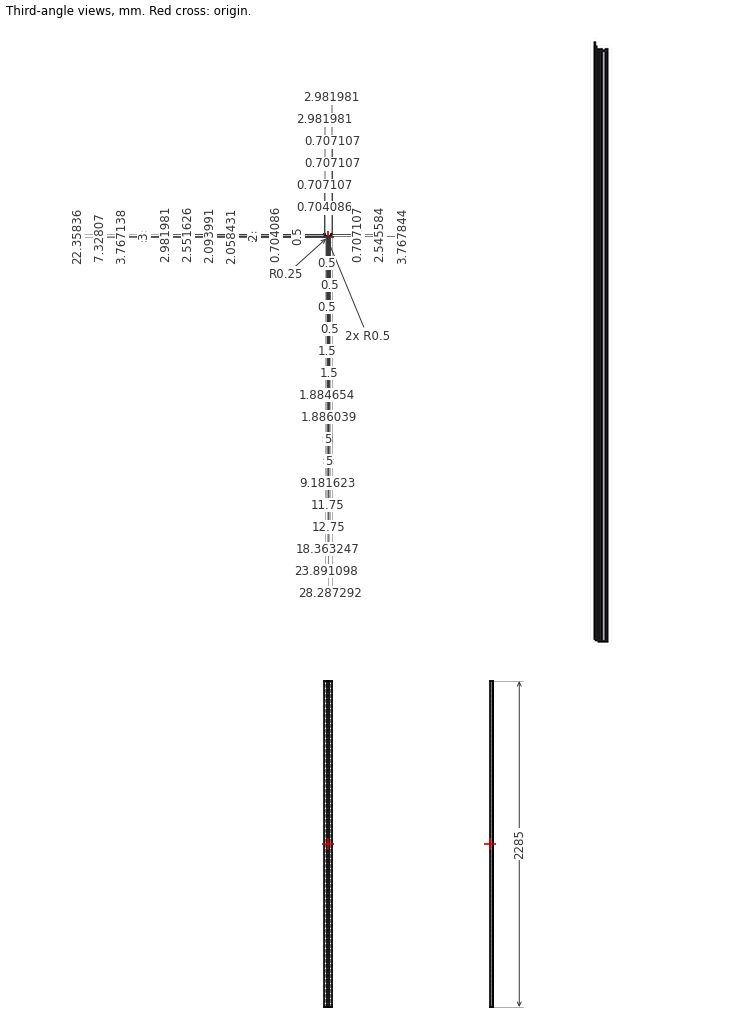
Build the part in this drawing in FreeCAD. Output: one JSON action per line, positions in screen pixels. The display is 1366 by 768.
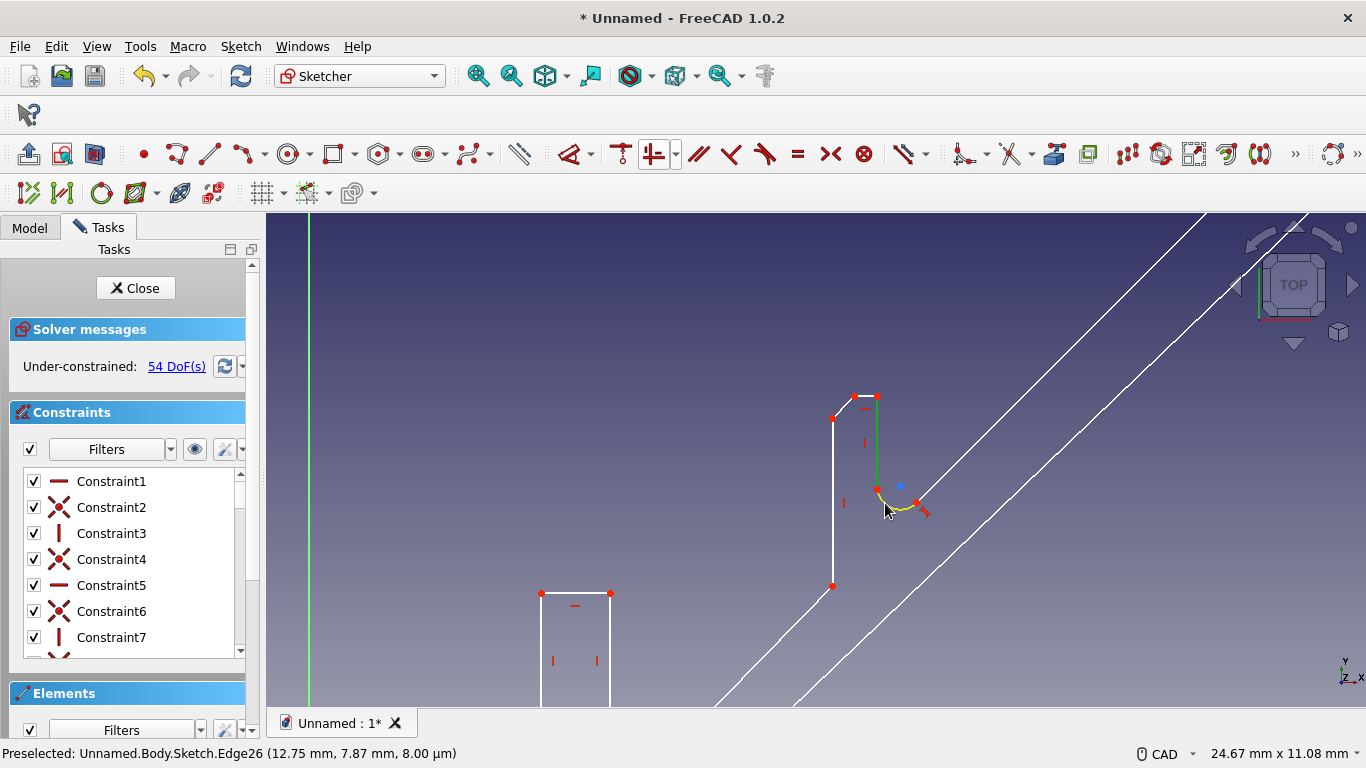
{"action": "left_click", "coordinate": [884, 503]}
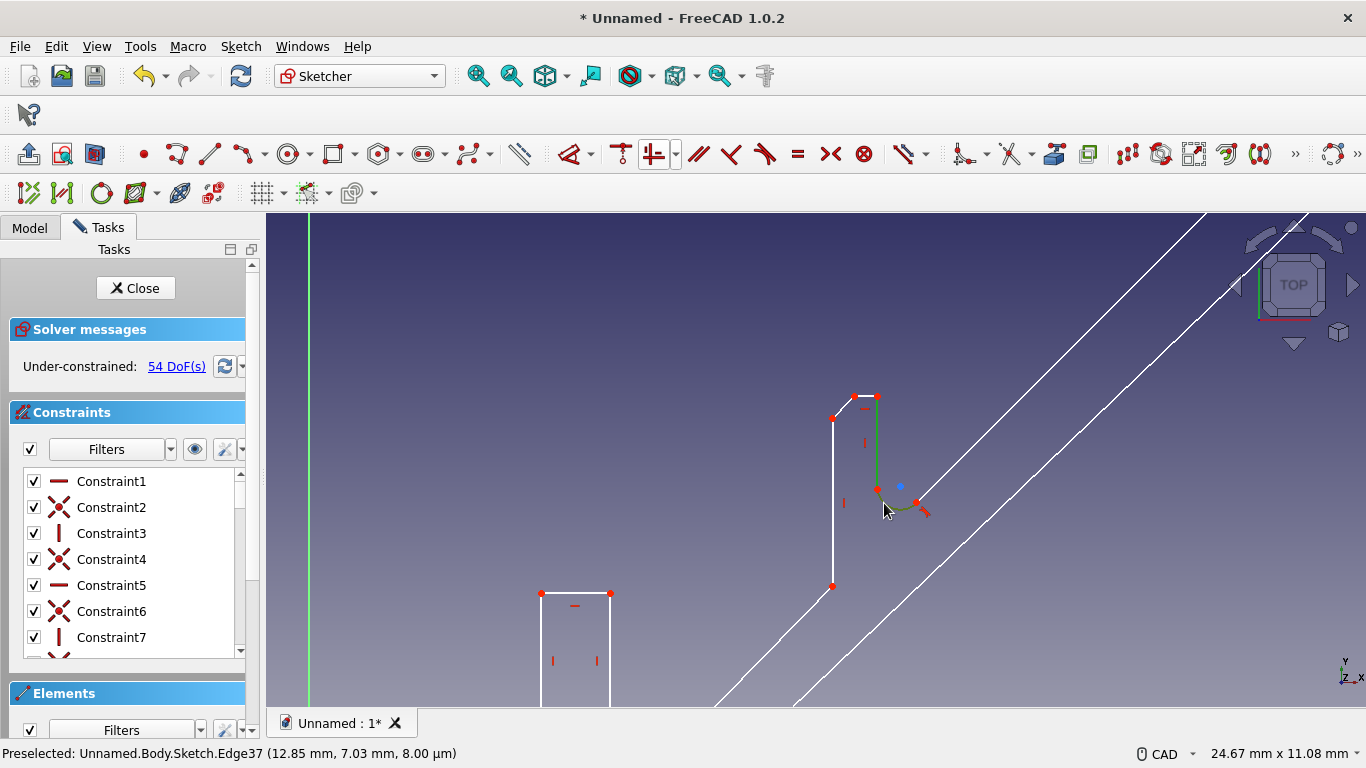
{"action": "left_click", "coordinate": [765, 154]}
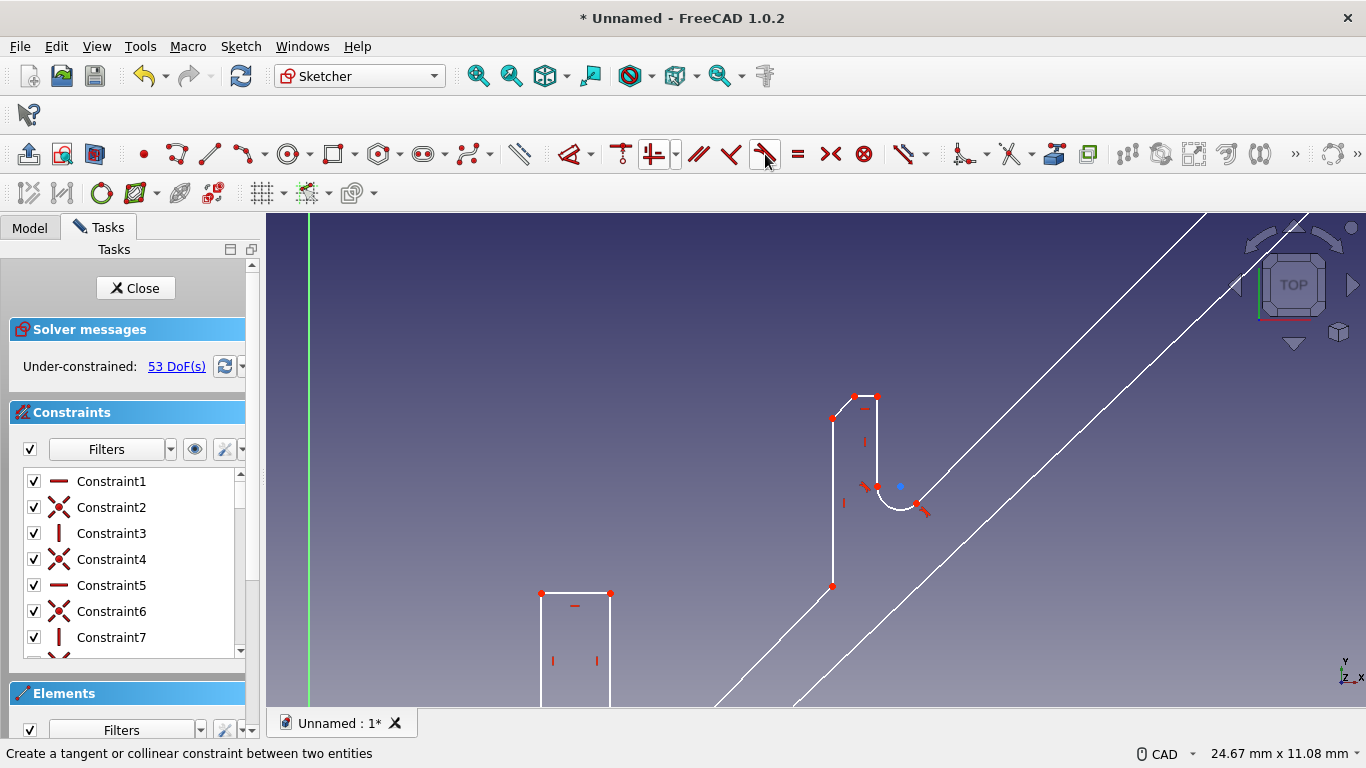
{"action": "scroll", "coordinate": [891, 508], "scroll_direction": "down", "scroll_amount": 7}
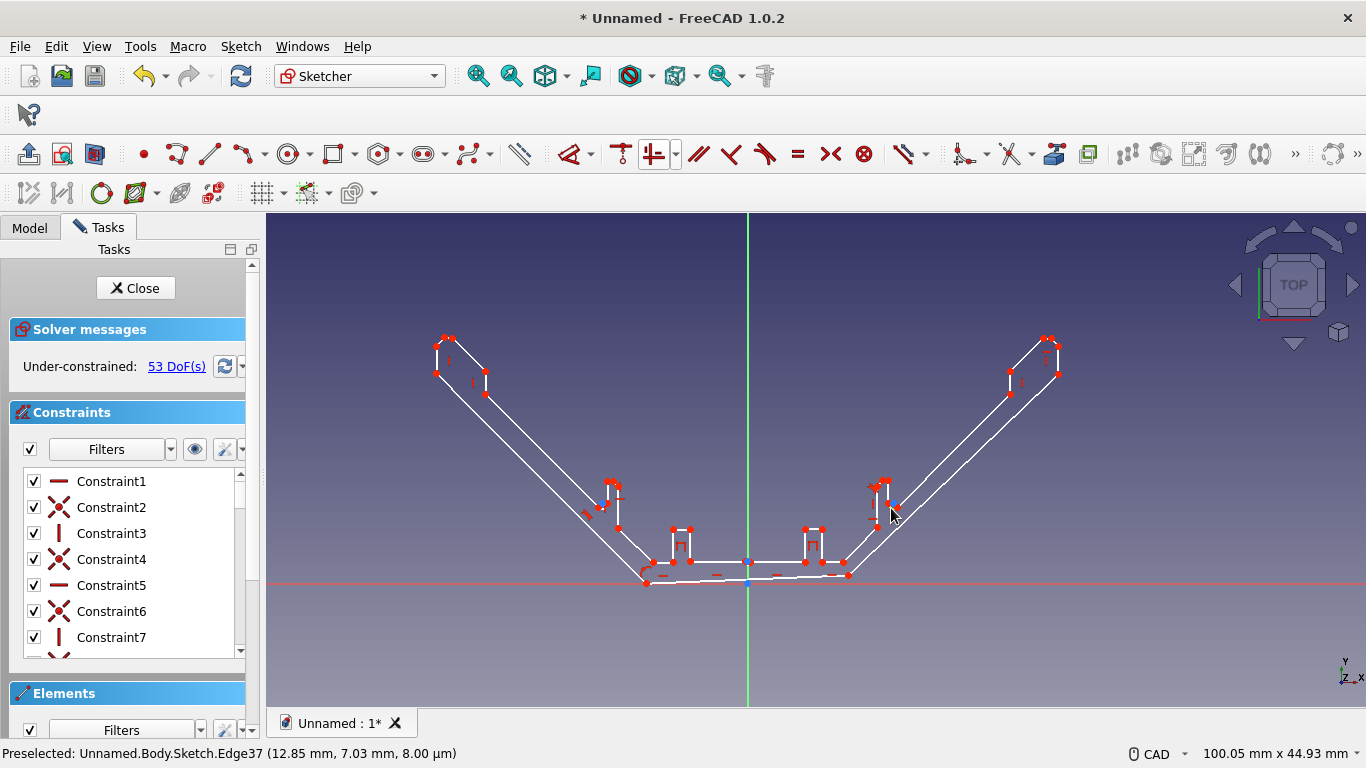
{"action": "scroll", "coordinate": [450, 338], "scroll_direction": "up", "scroll_amount": 9}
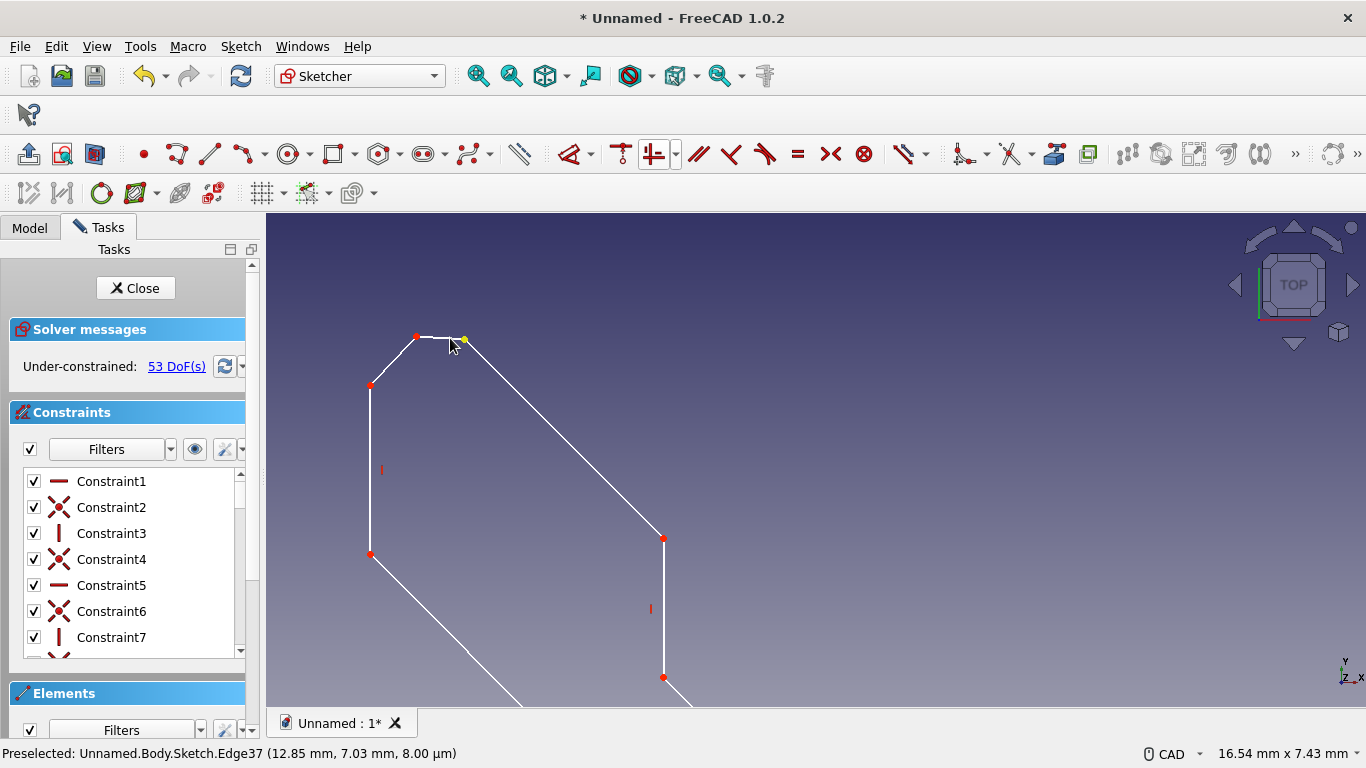
{"action": "left_click", "coordinate": [450, 338]}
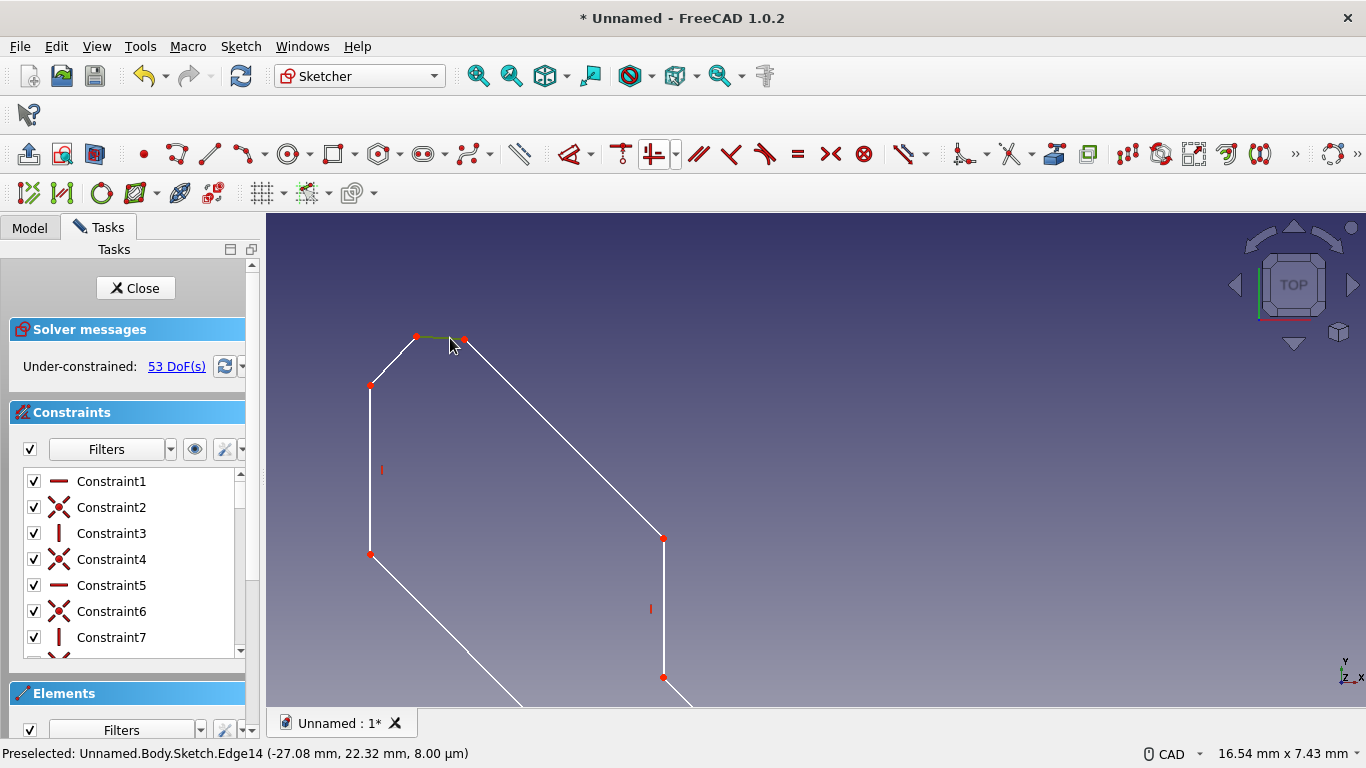
{"action": "left_click", "coordinate": [676, 154]}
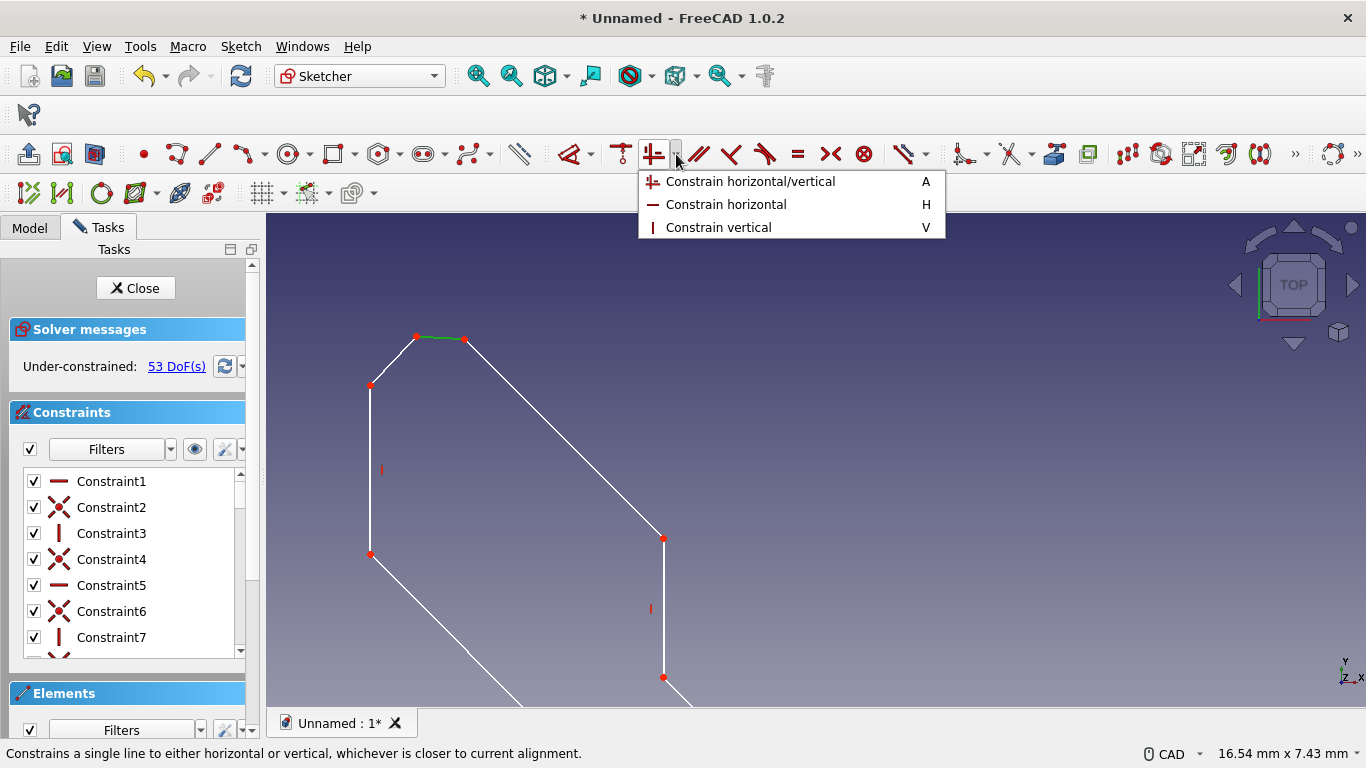
{"action": "left_click", "coordinate": [792, 204]}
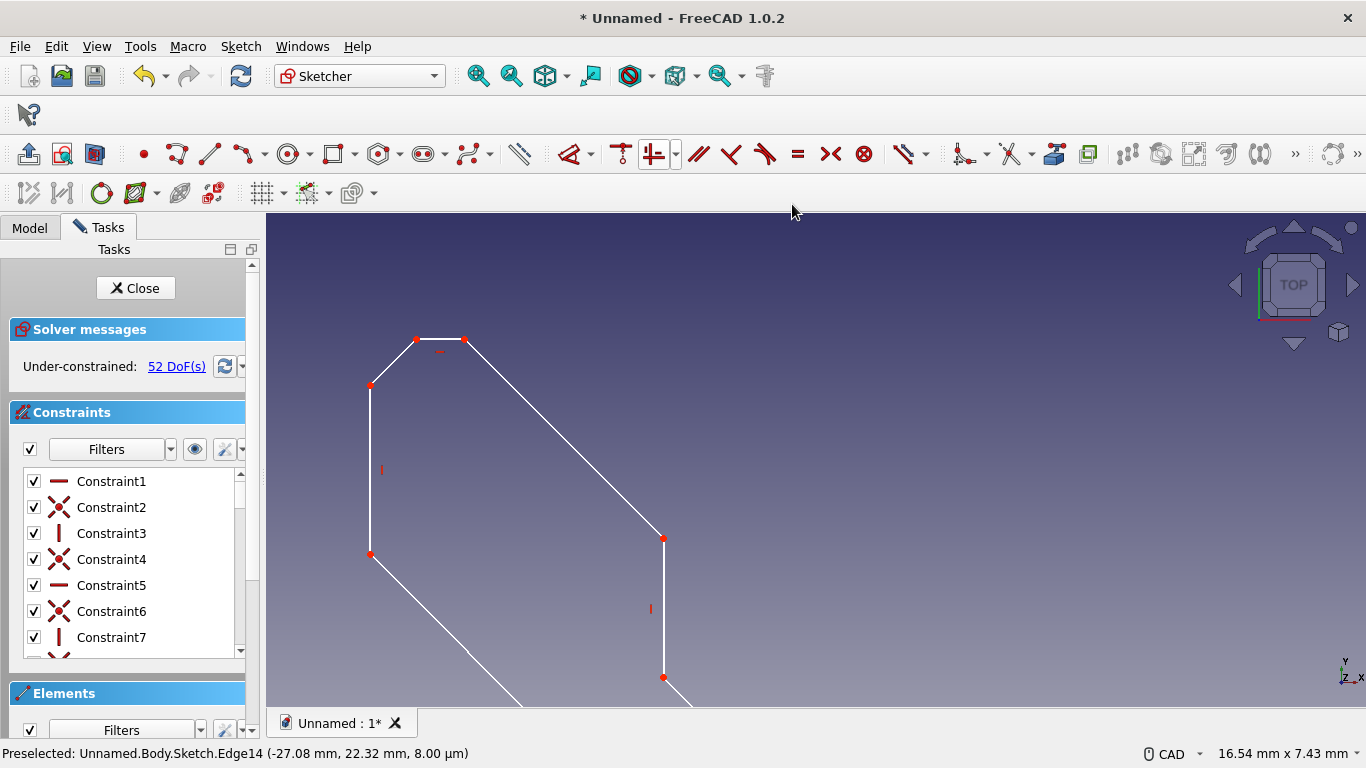
{"action": "scroll", "coordinate": [450, 337], "scroll_direction": "down", "scroll_amount": 9}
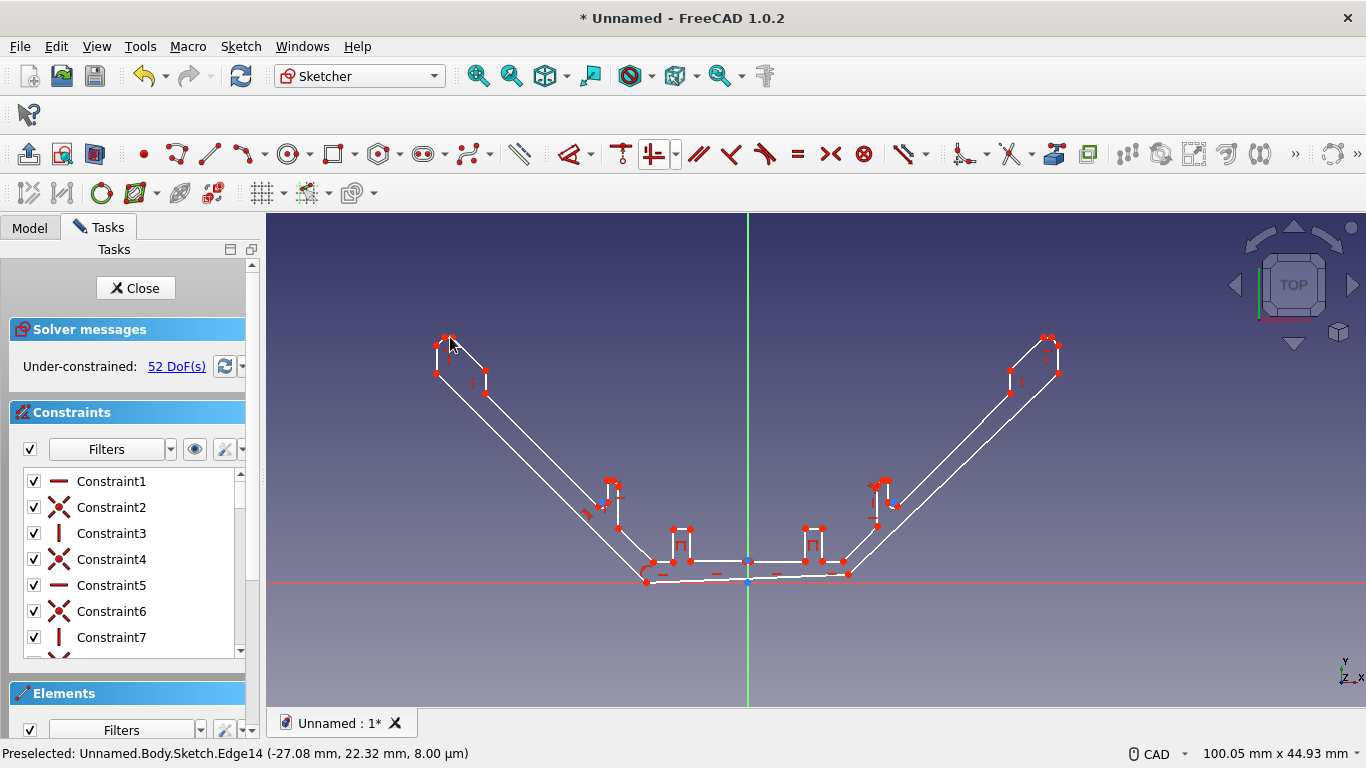
{"action": "scroll", "coordinate": [707, 580], "scroll_direction": "up", "scroll_amount": 9}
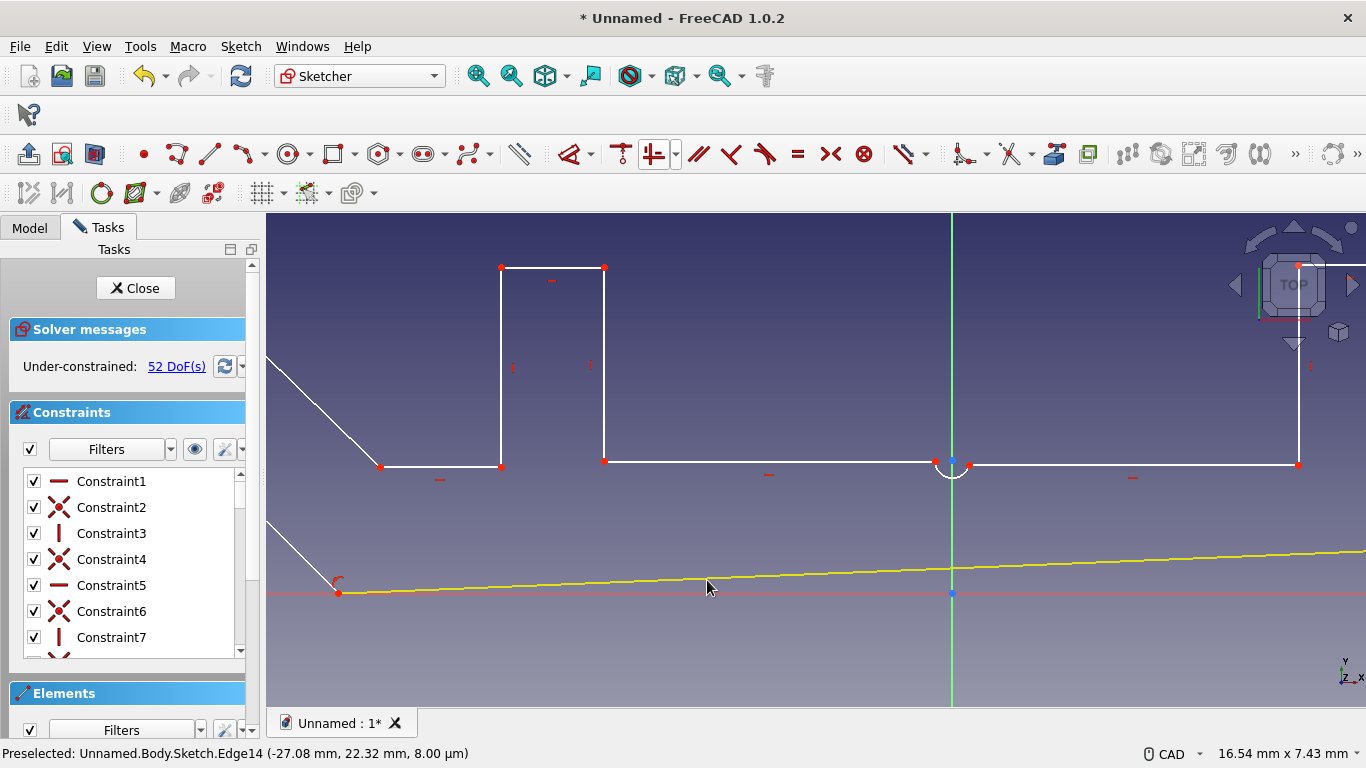
{"action": "left_click", "coordinate": [706, 579]}